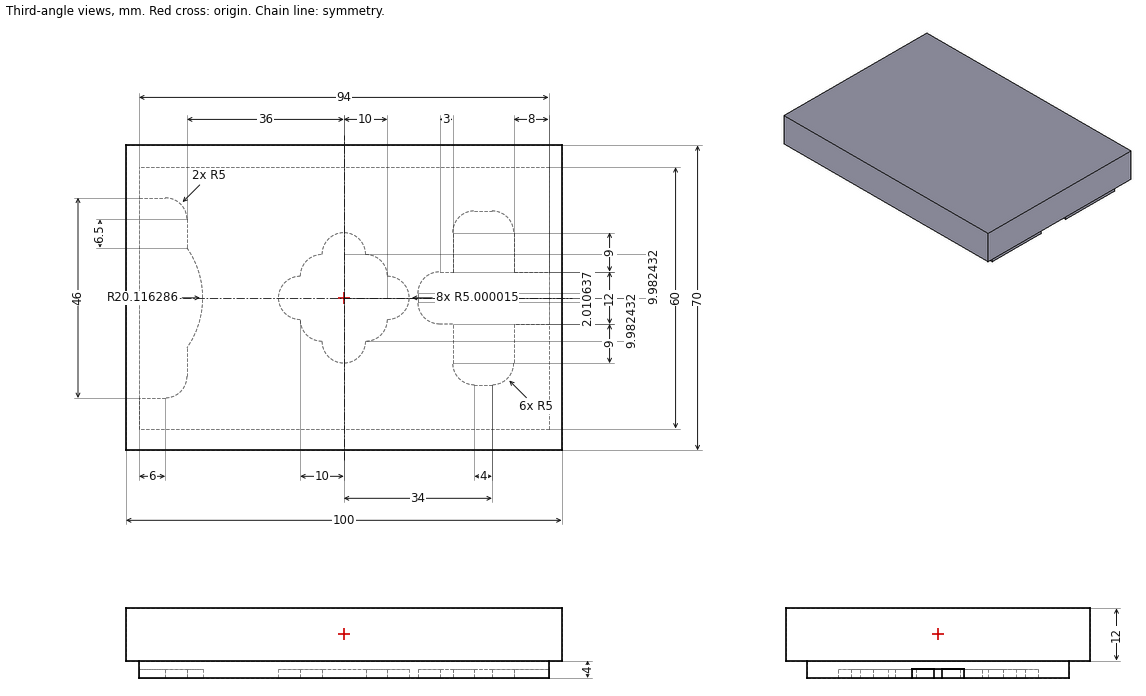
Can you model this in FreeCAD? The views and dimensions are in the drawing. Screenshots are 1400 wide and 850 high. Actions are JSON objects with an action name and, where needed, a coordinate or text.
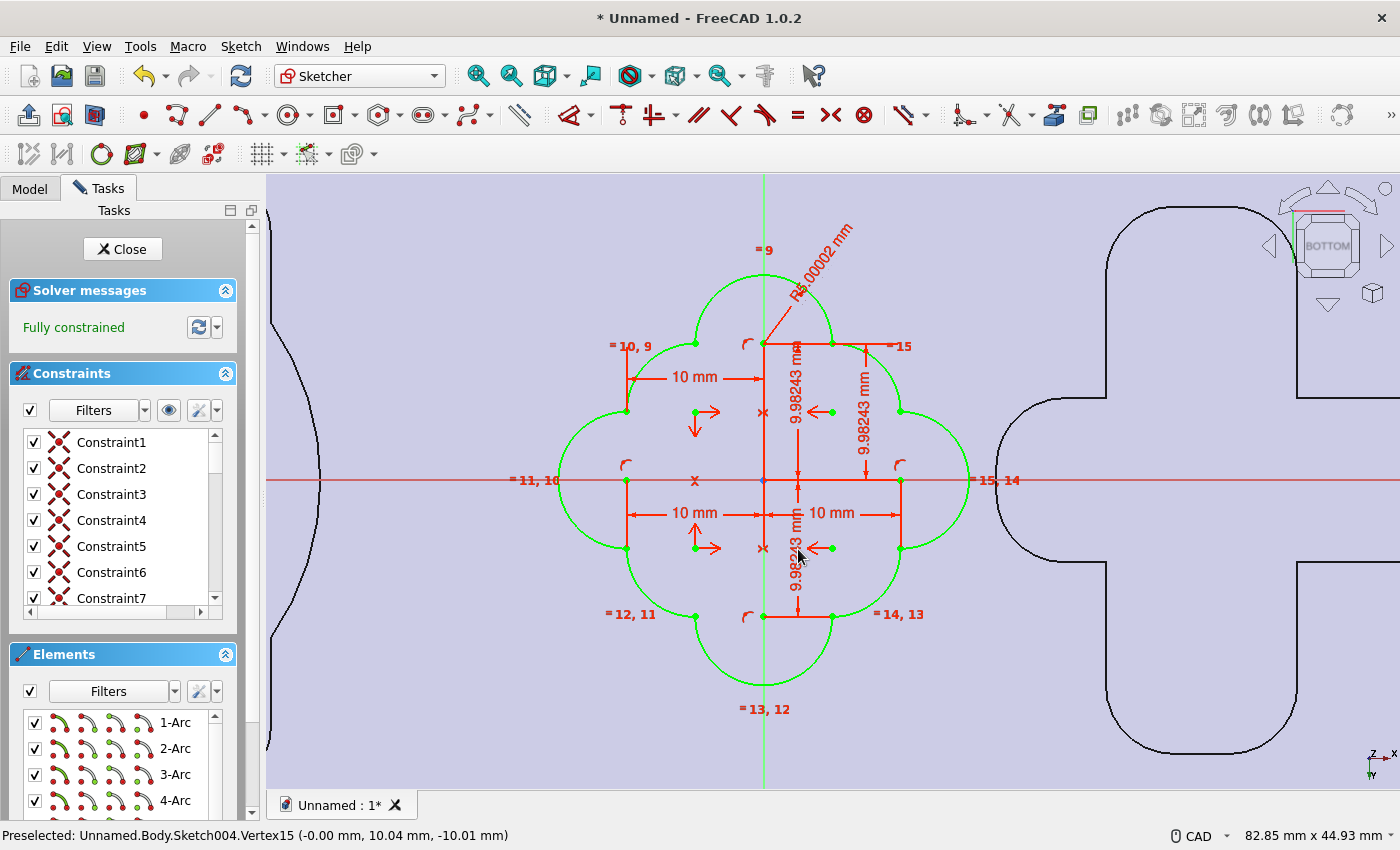
{"action": "left_click", "coordinate": [123, 249]}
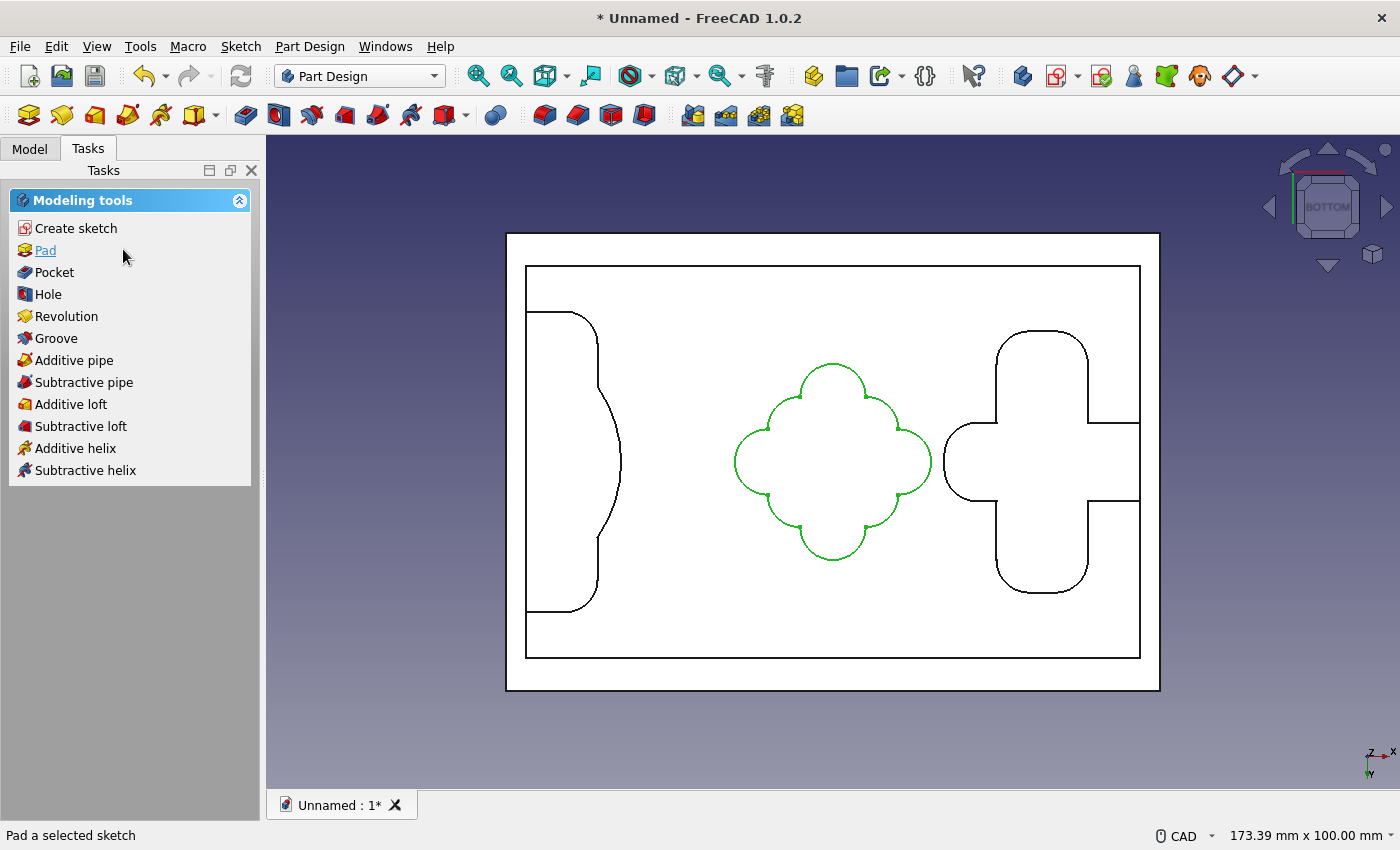
{"action": "left_click", "coordinate": [246, 116]}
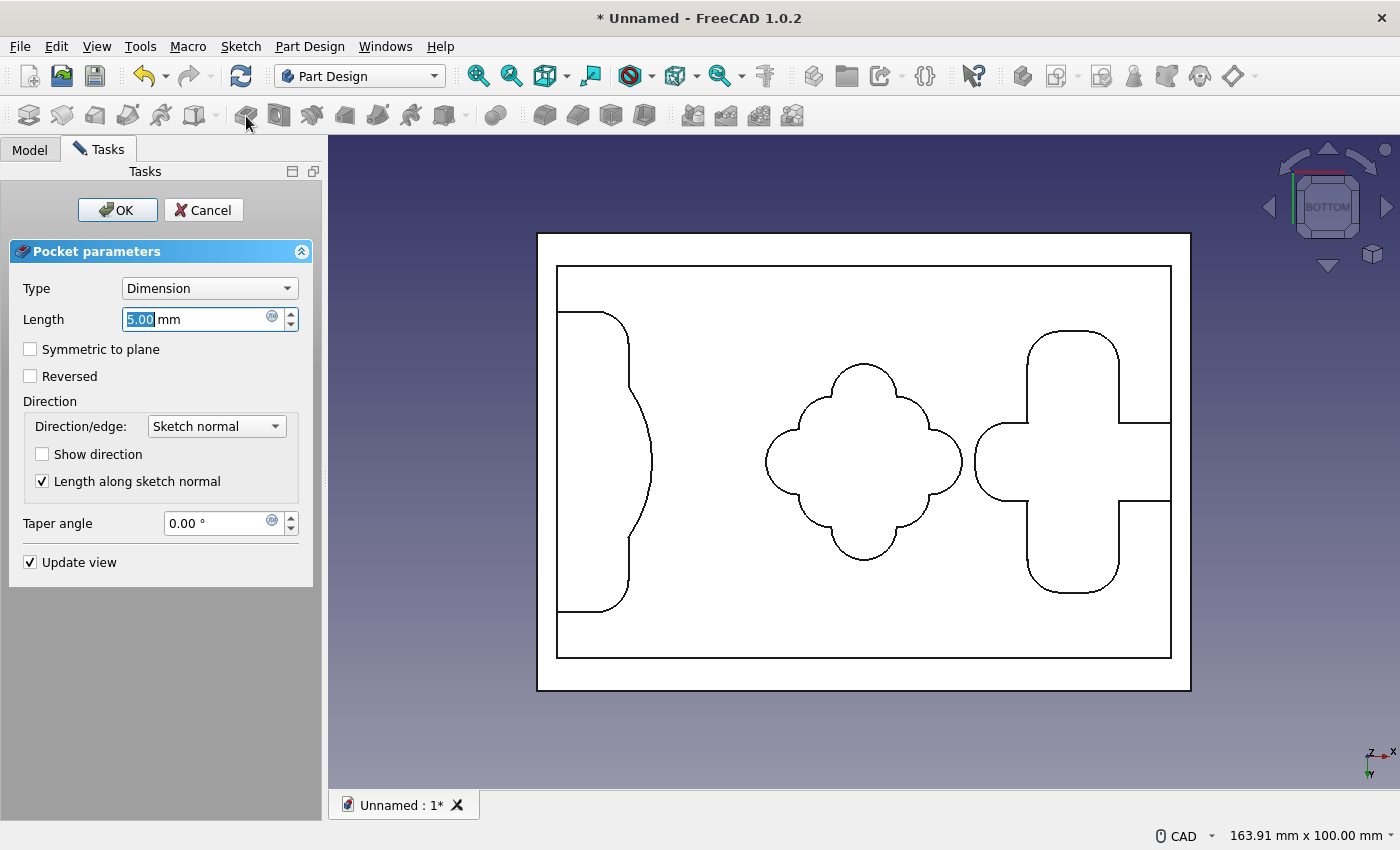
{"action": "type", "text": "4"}
{"action": "key", "text": "Tab"}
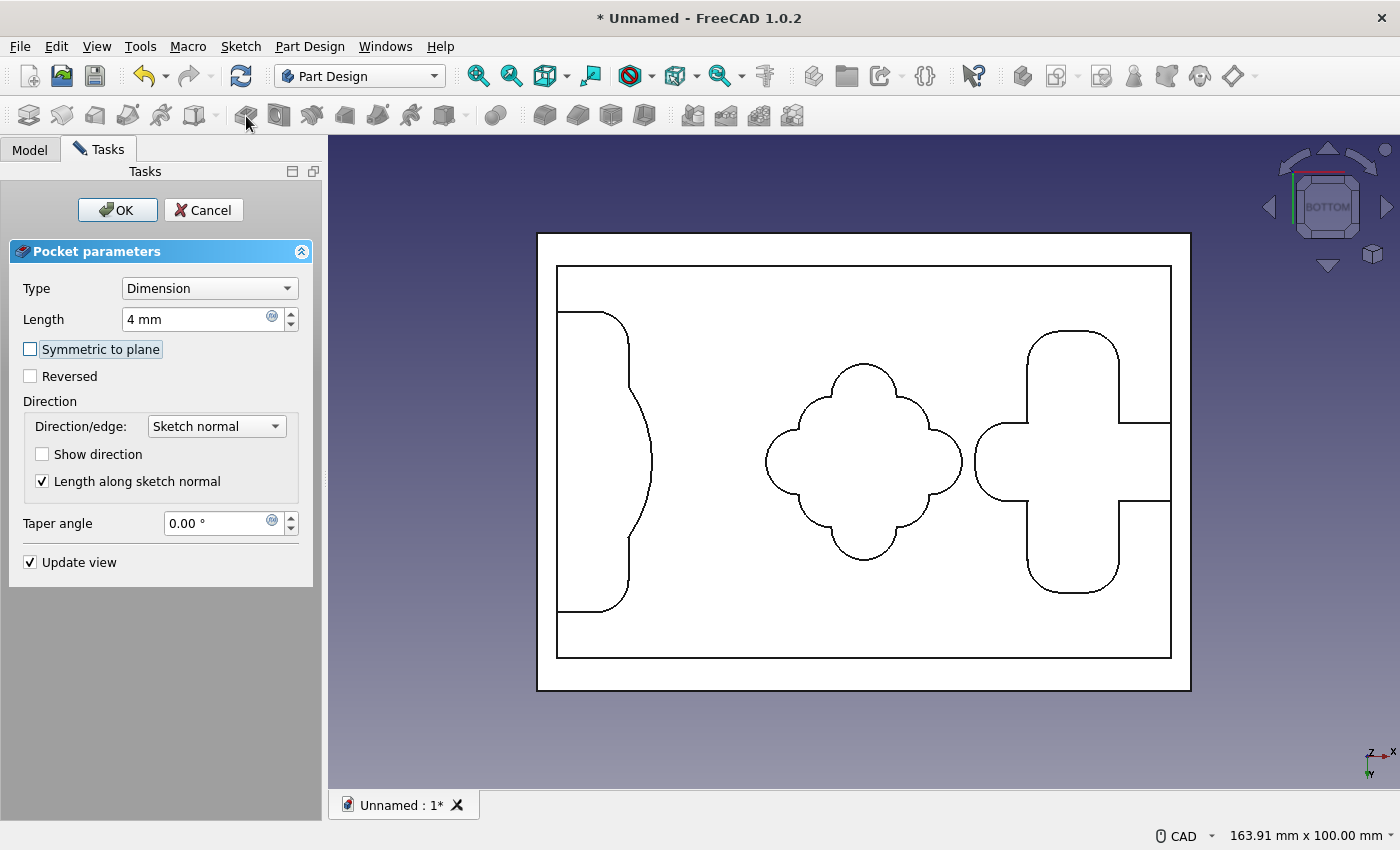
{"action": "left_click", "coordinate": [31, 349]}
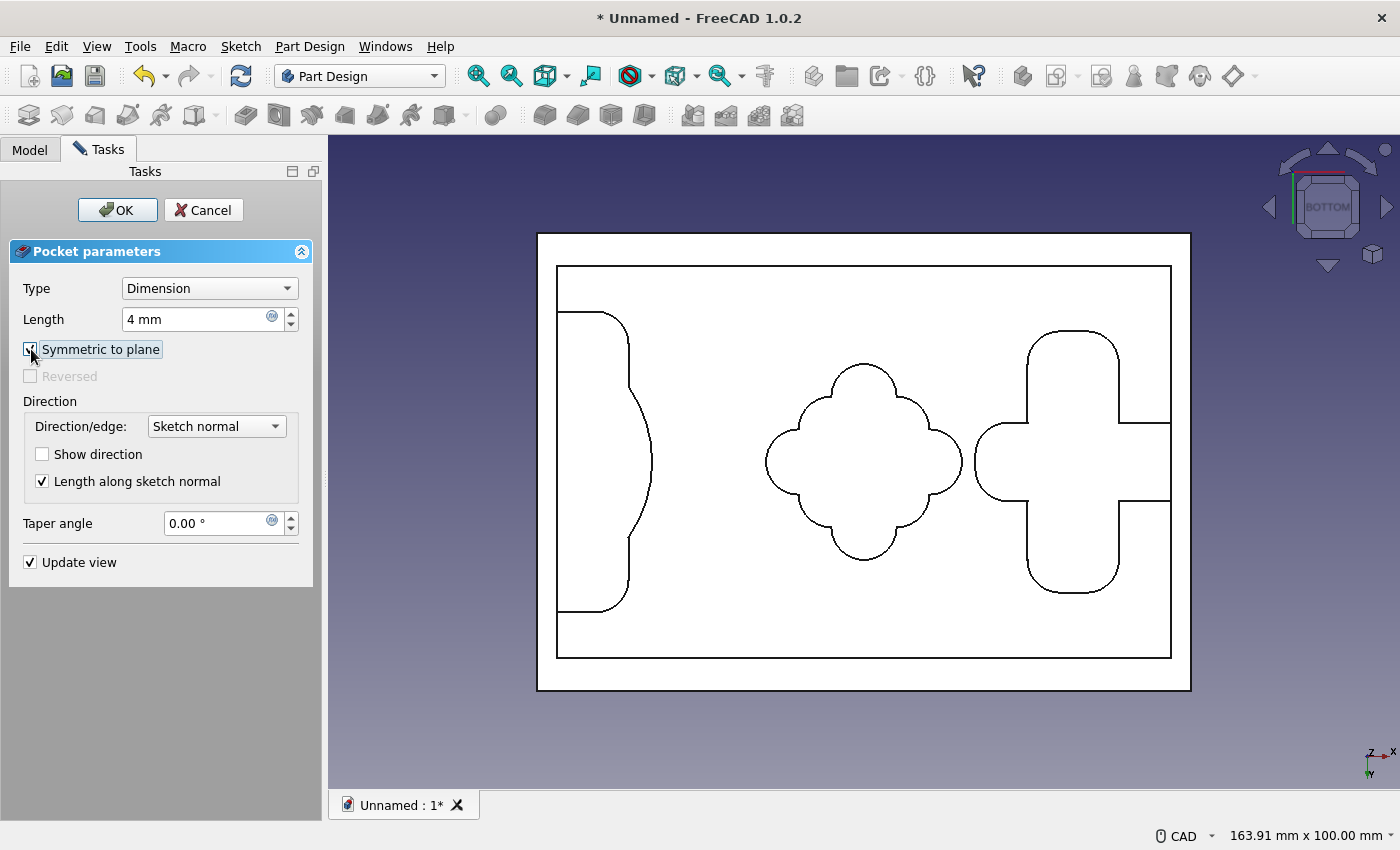
{"action": "left_click", "coordinate": [118, 210]}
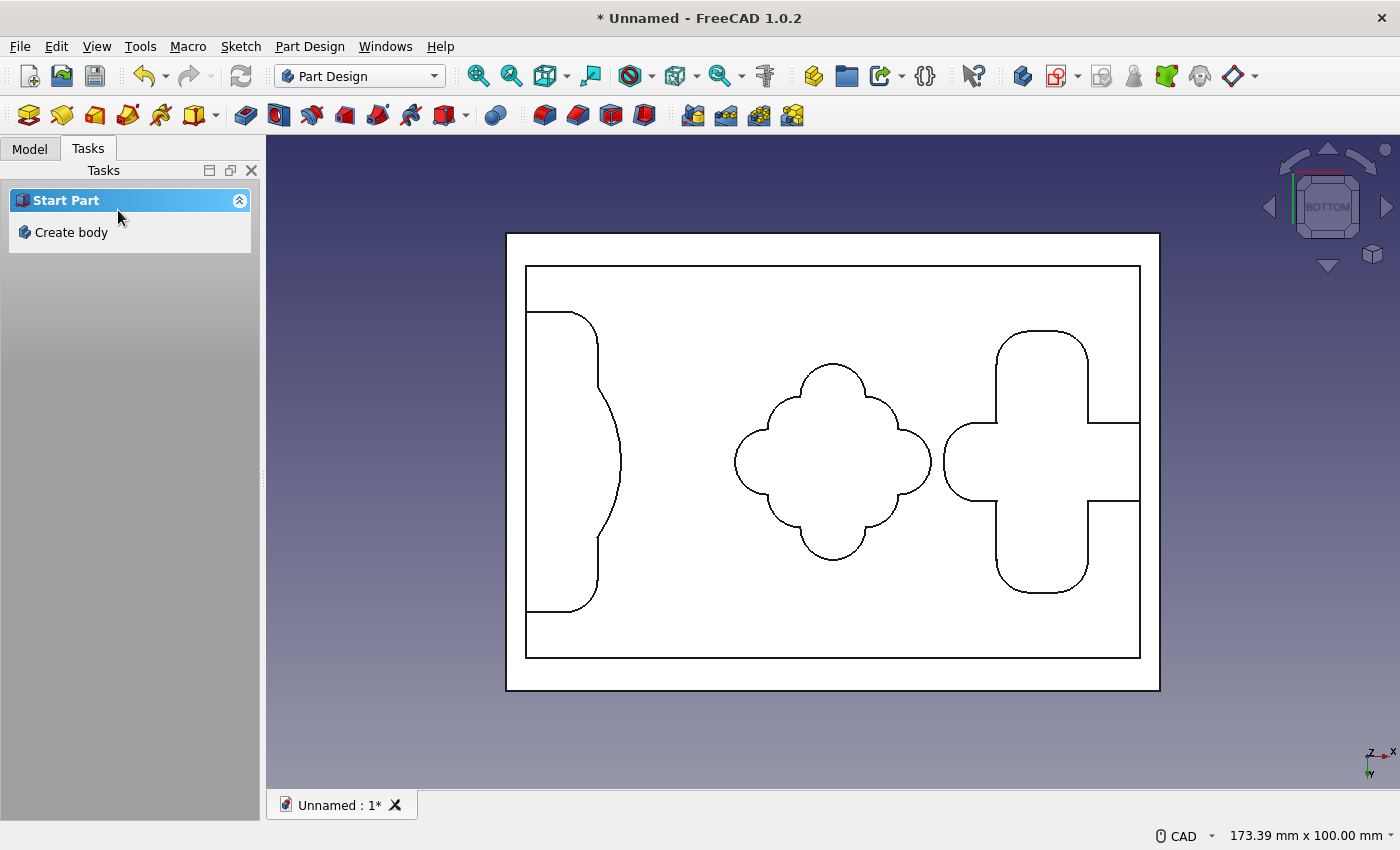
{"action": "key", "text": "0"}